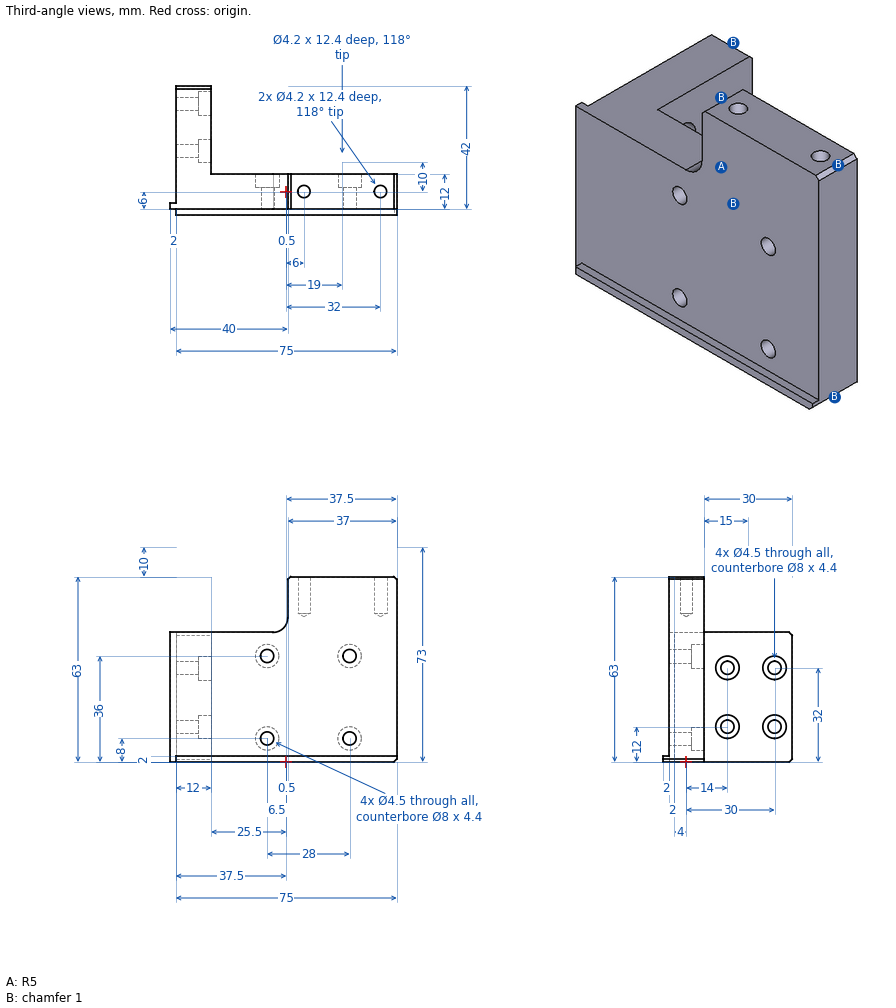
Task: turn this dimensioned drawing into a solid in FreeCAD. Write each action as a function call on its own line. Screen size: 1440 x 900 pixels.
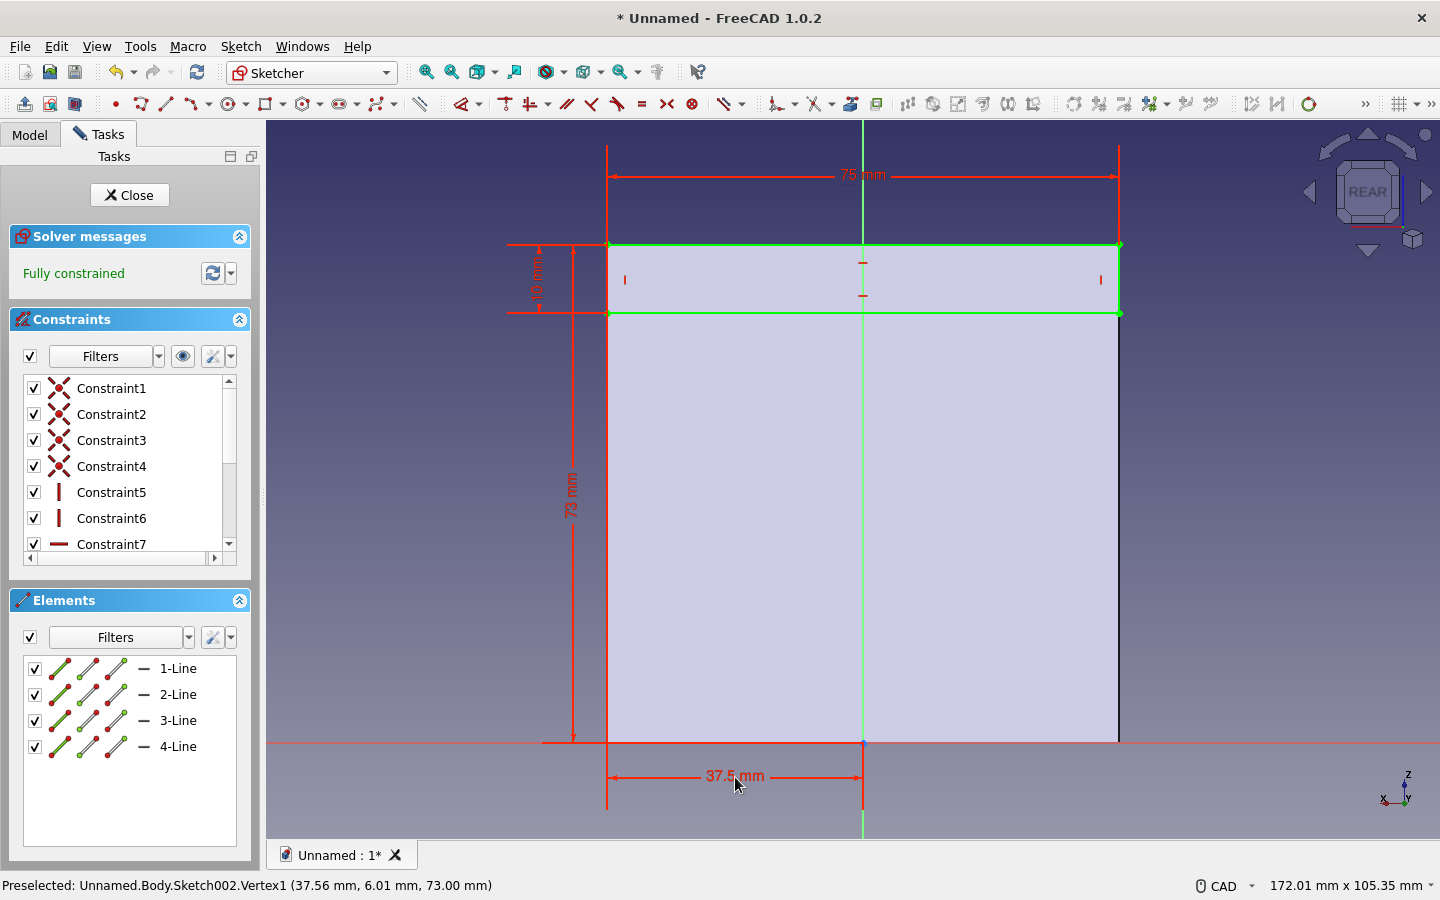
click(130, 195)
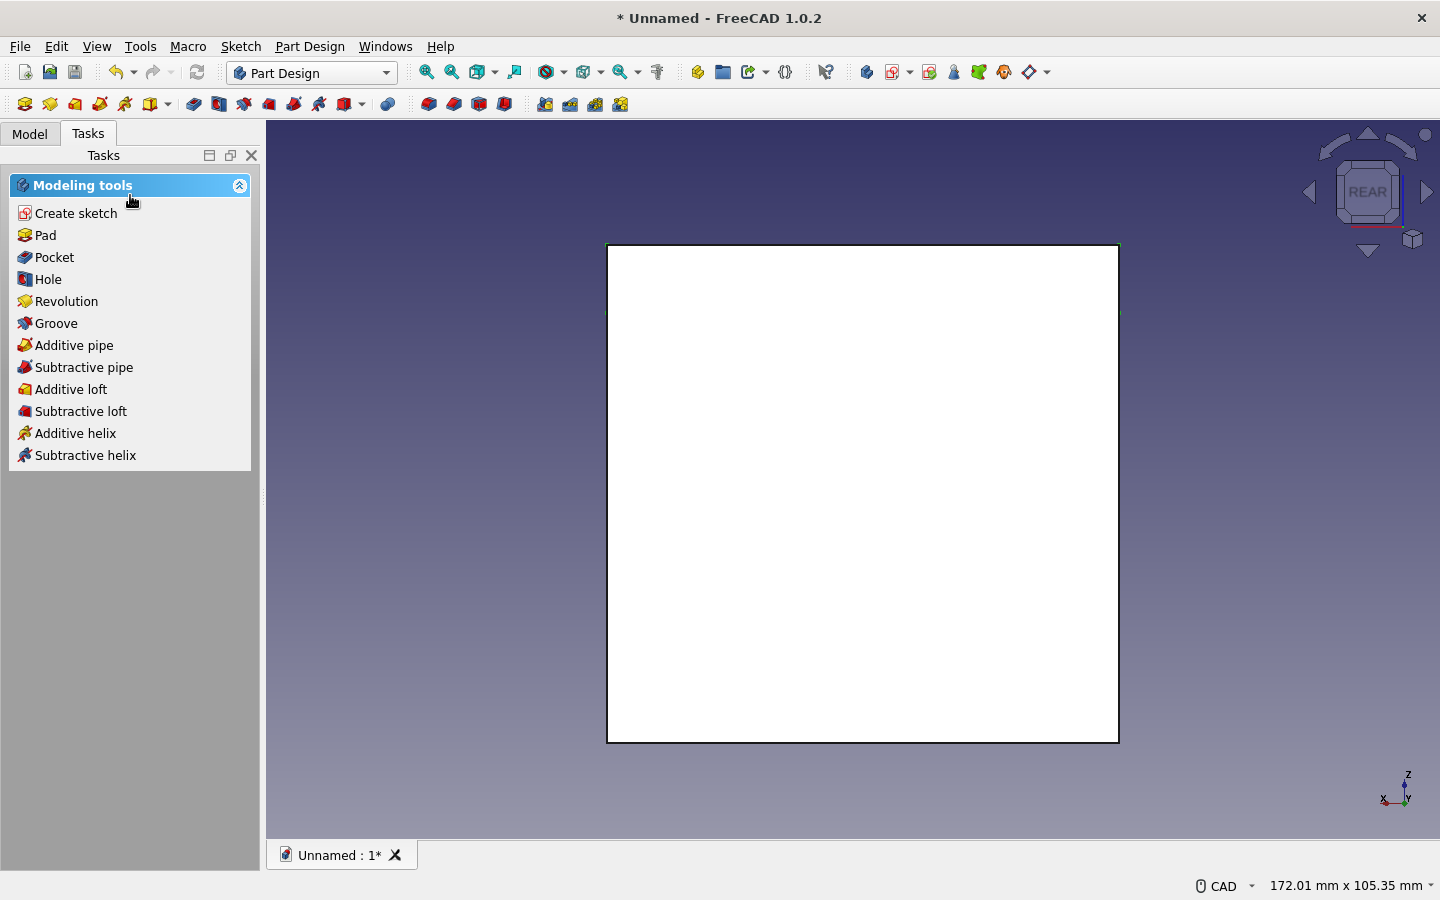
click(25, 104)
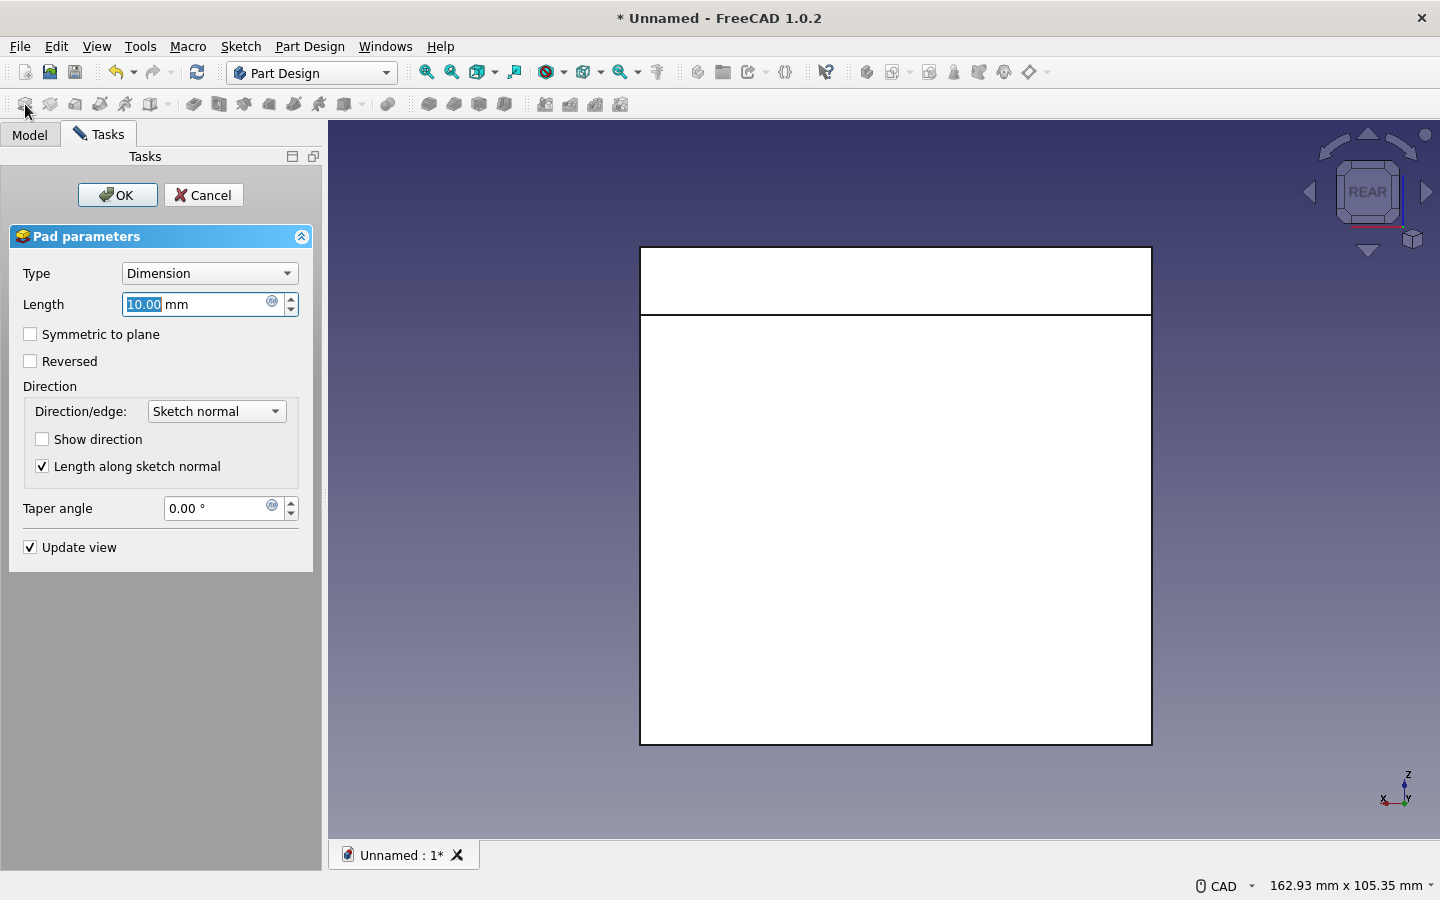
text(15)
key(Tab)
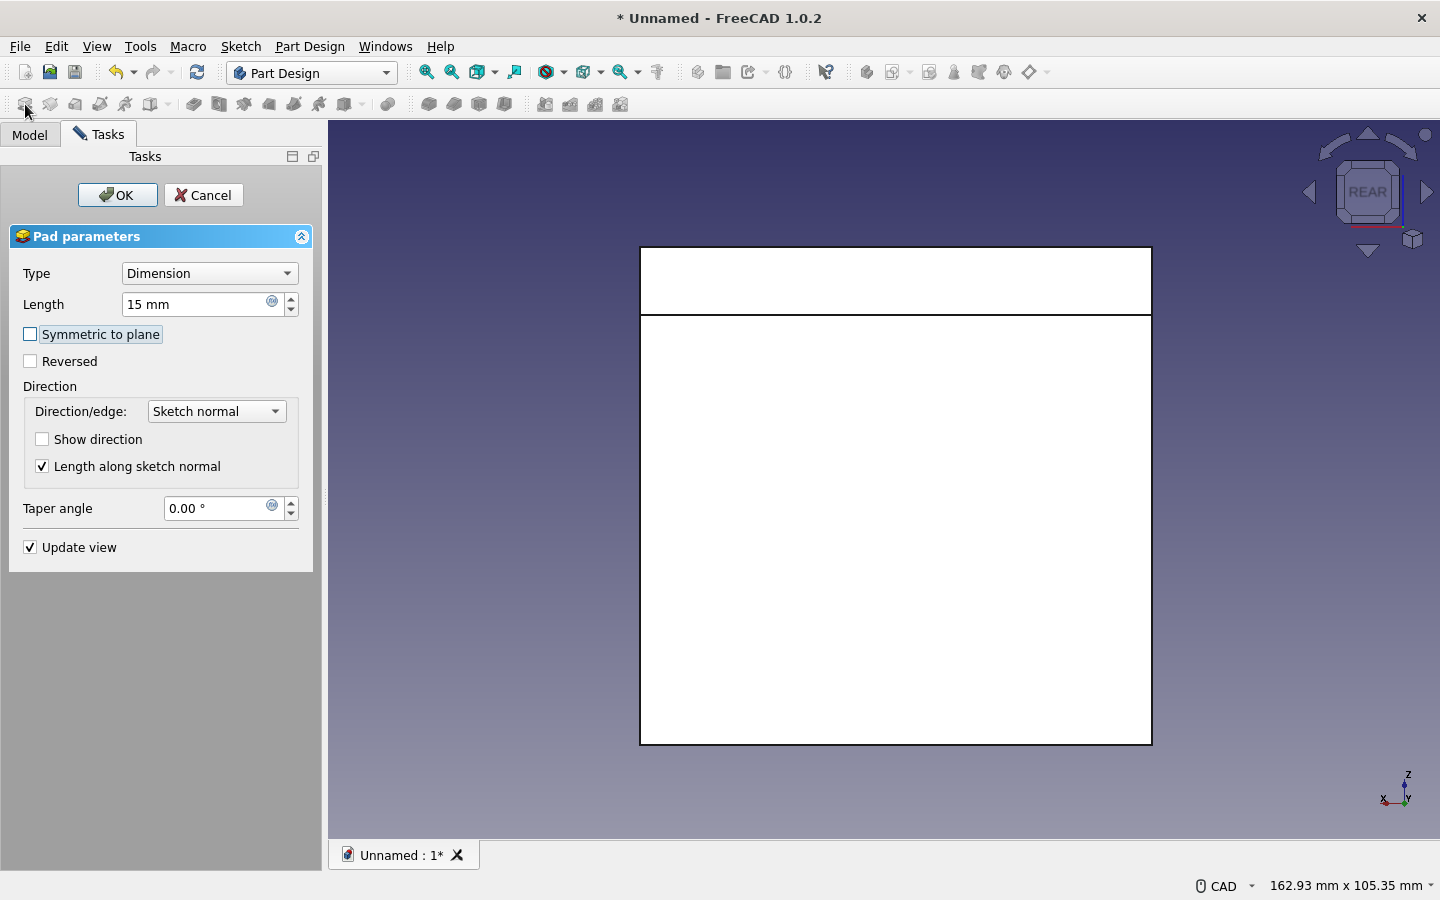
click(118, 195)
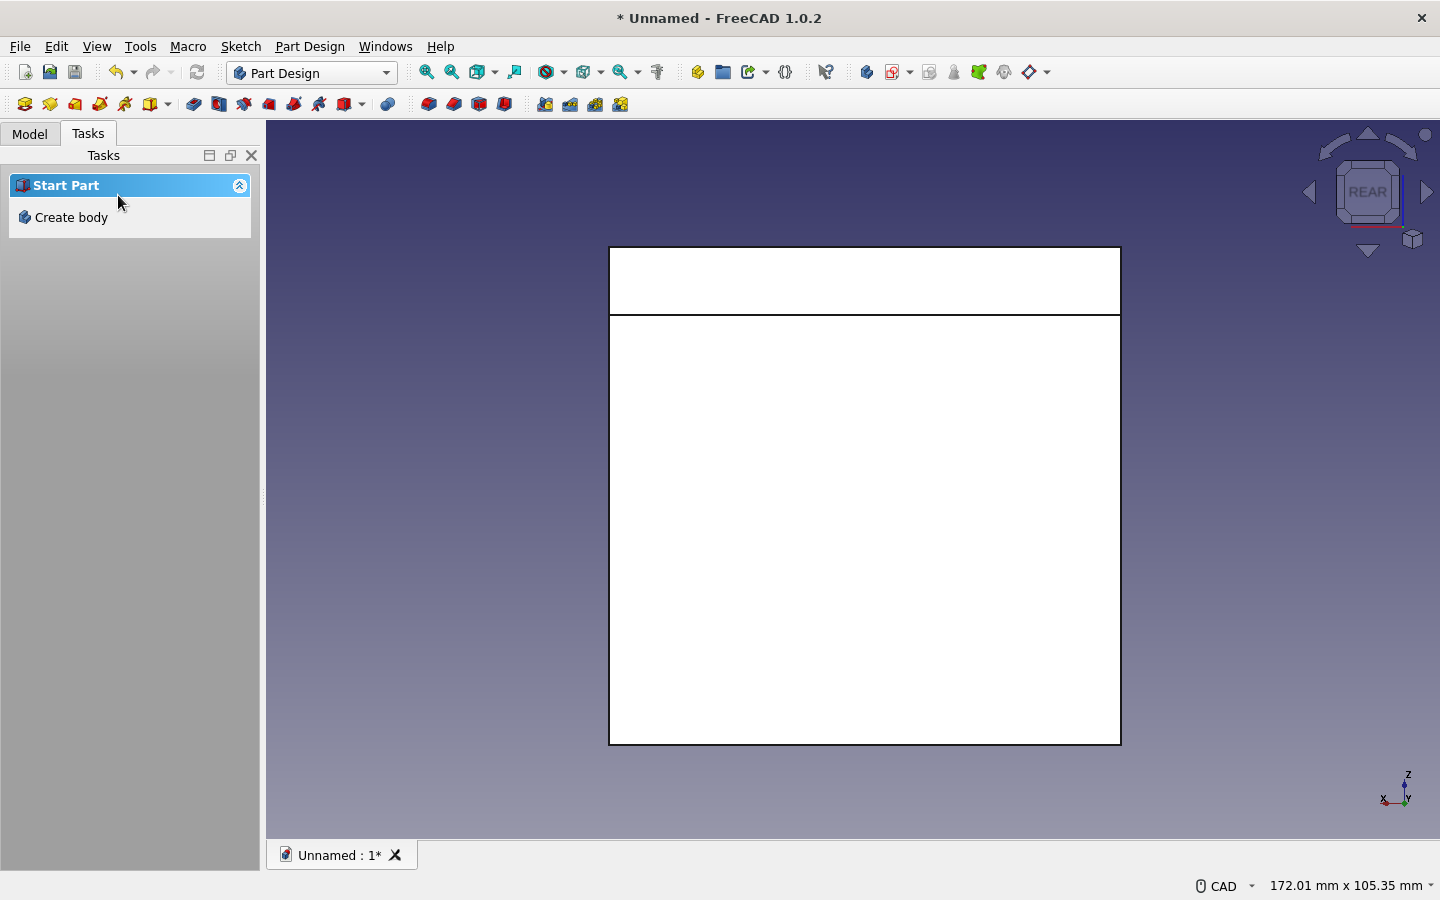
click(865, 529)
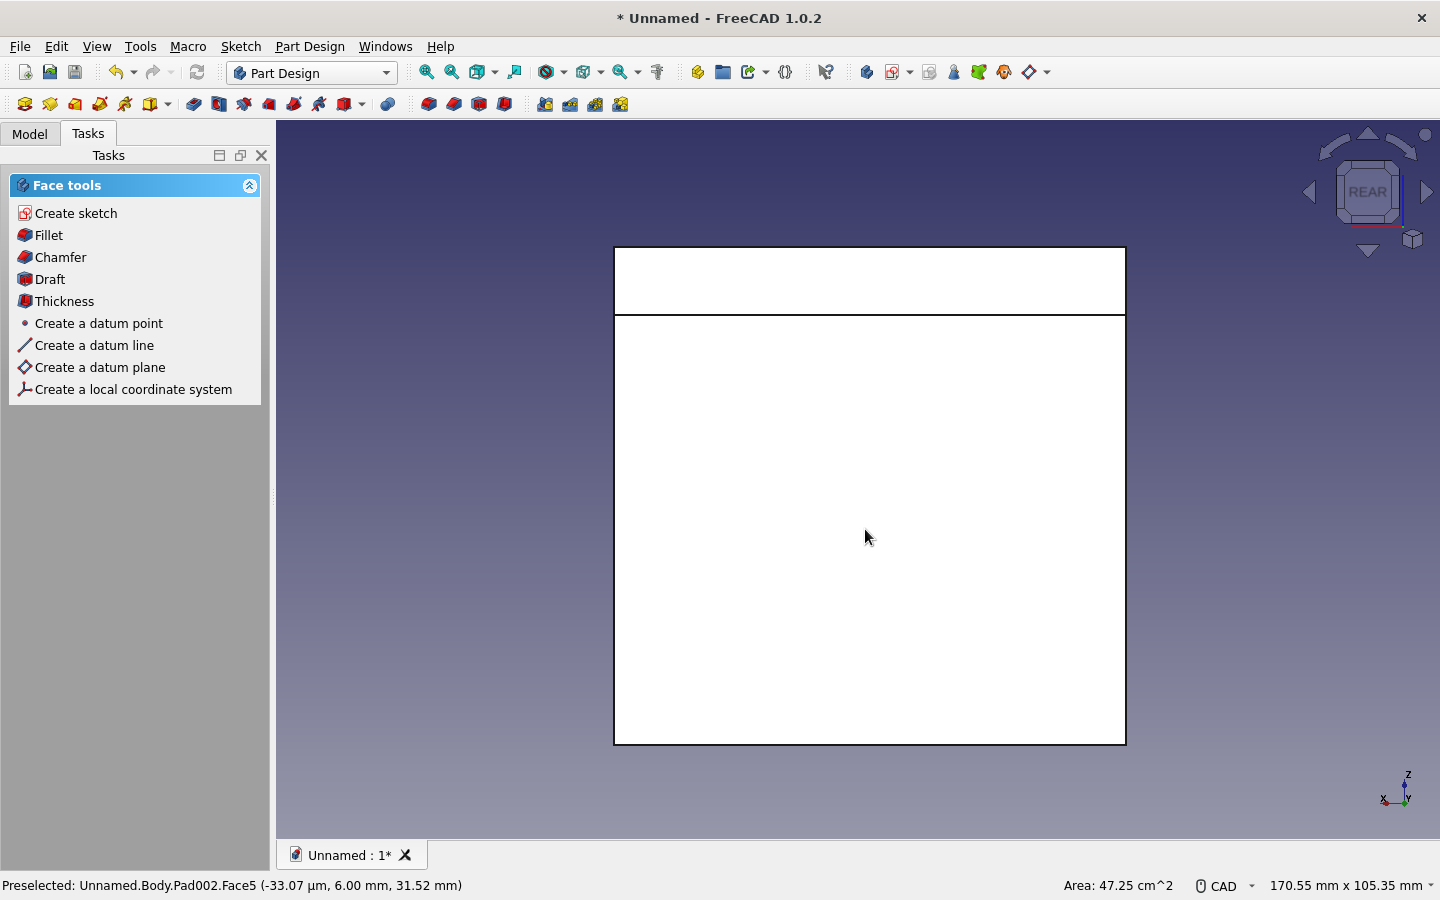
click(892, 72)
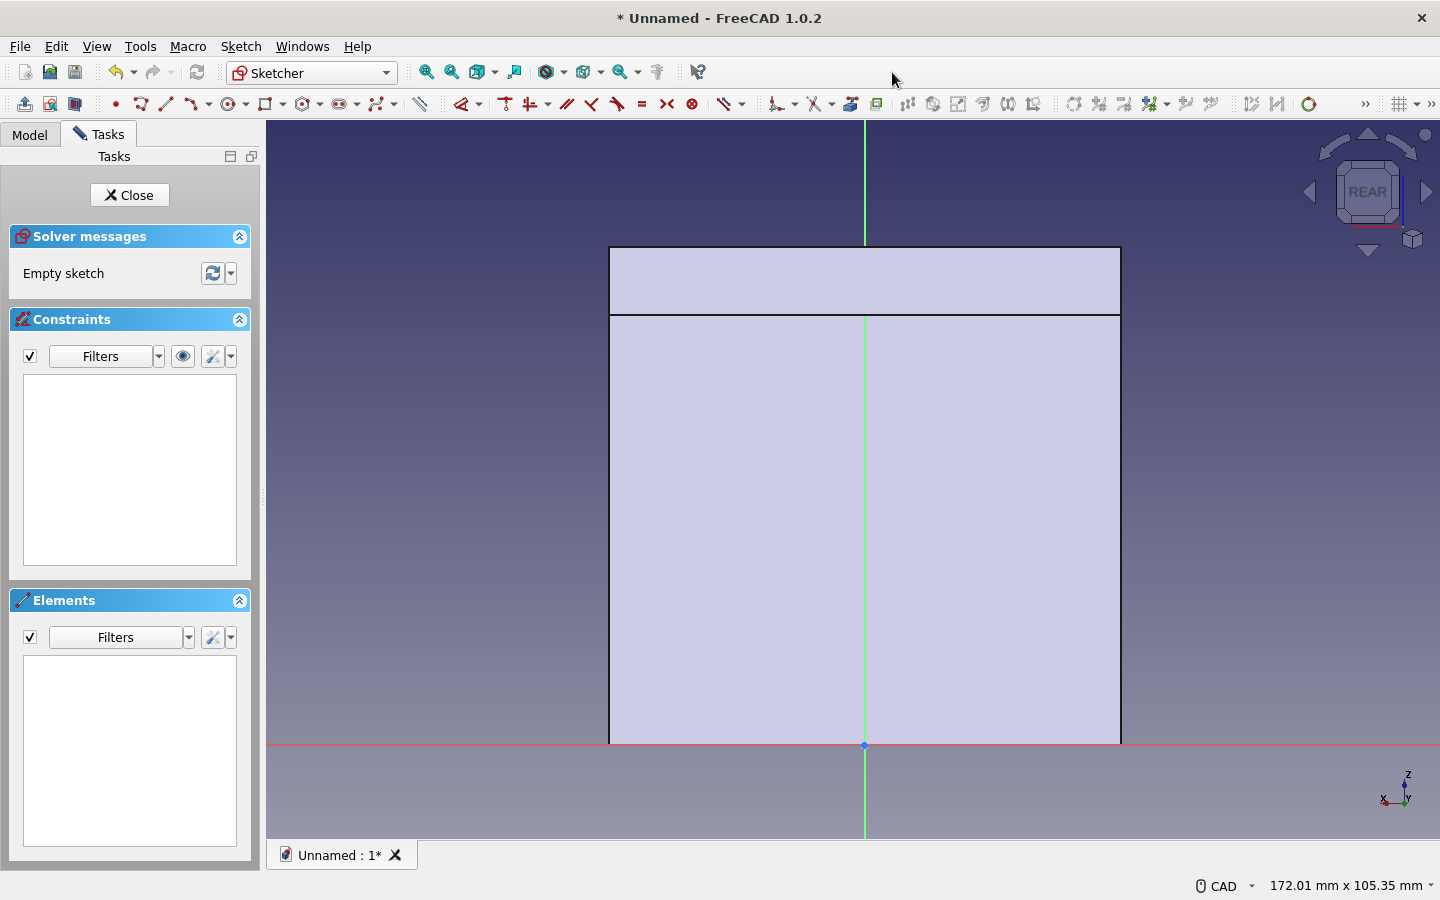
click(264, 104)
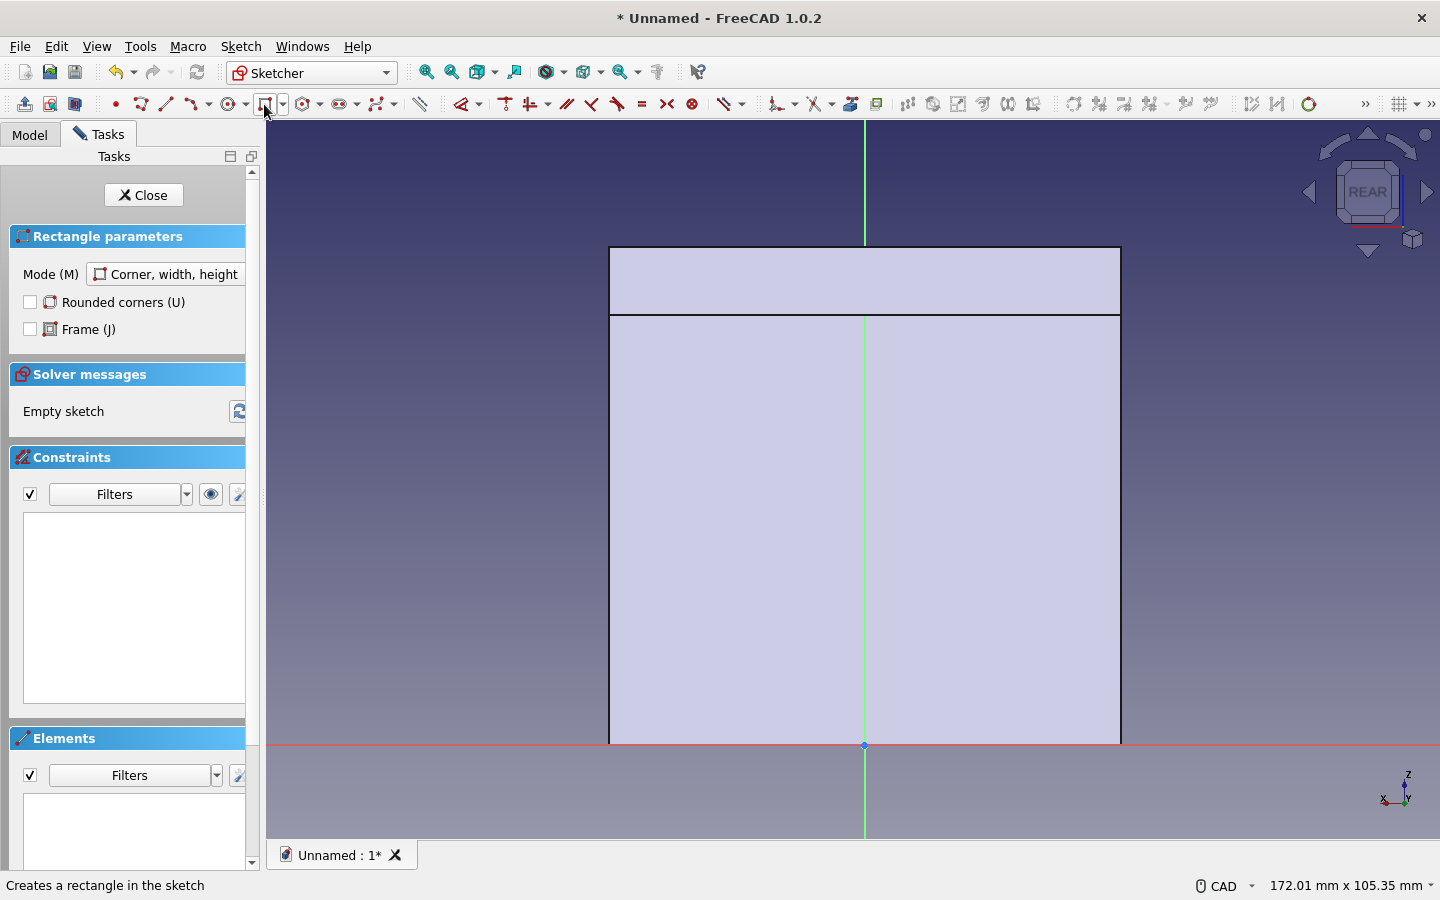
click(1039, 315)
click(1121, 745)
key(Escape)